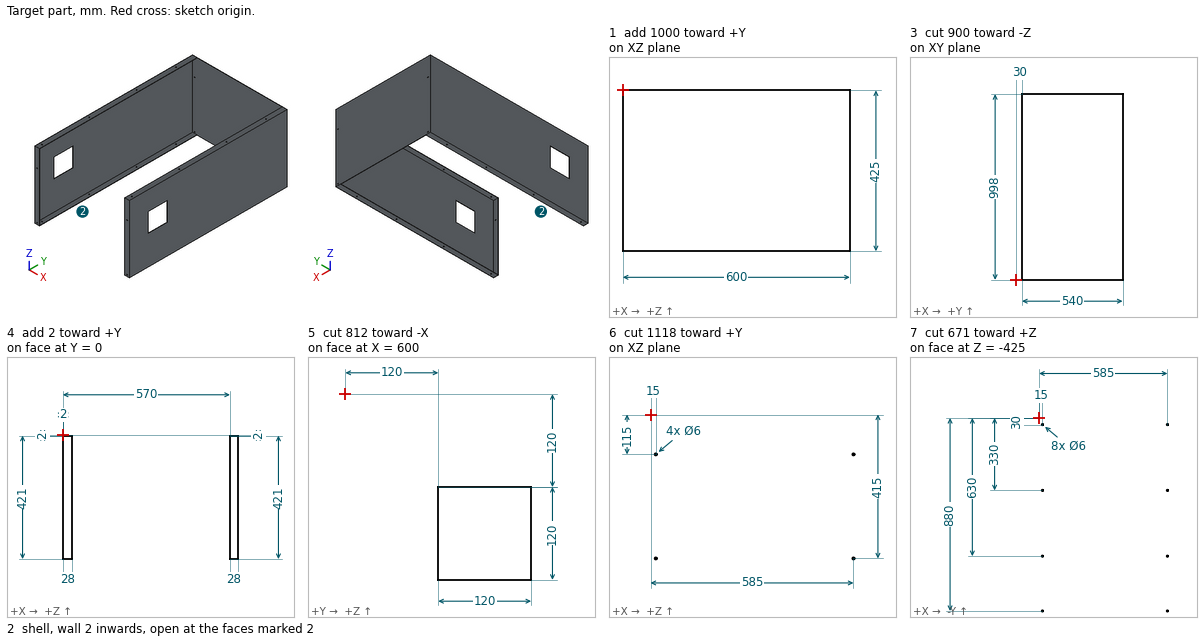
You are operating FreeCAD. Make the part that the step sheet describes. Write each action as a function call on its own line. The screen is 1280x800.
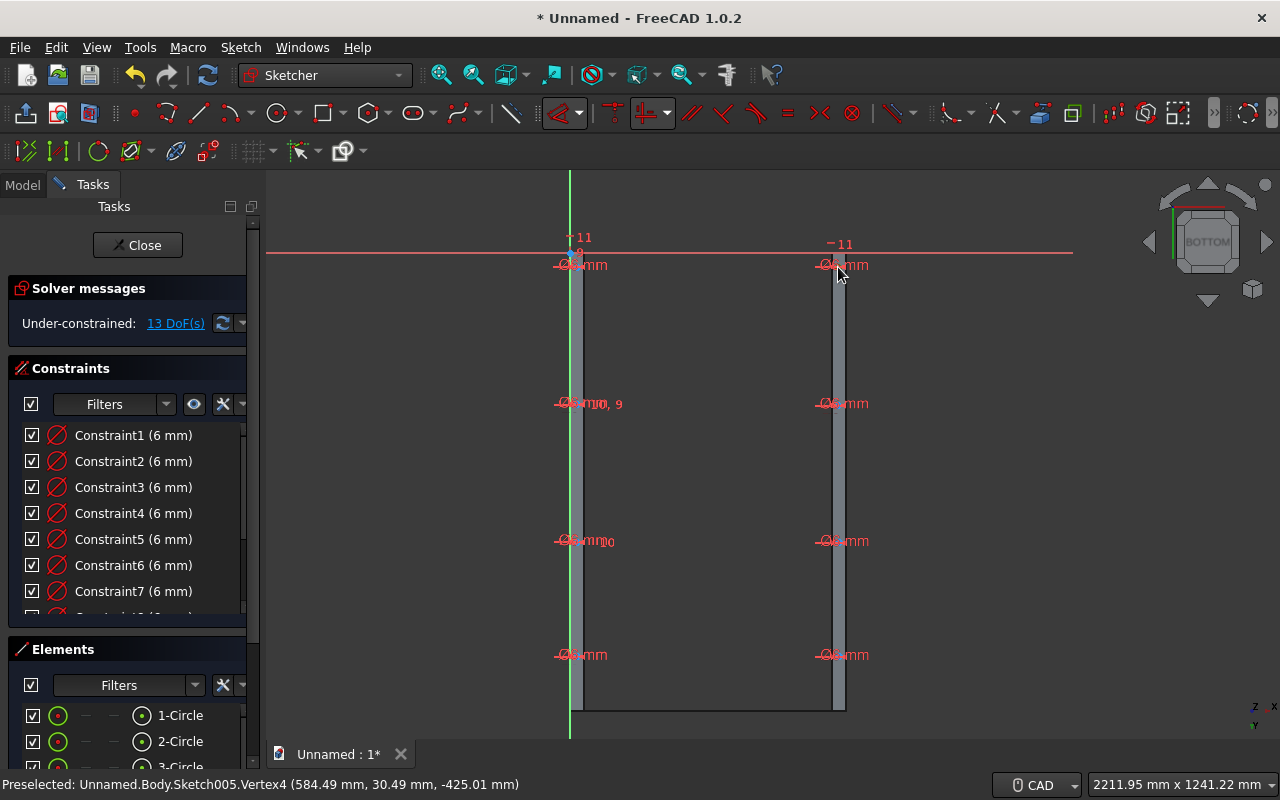
click(838, 406)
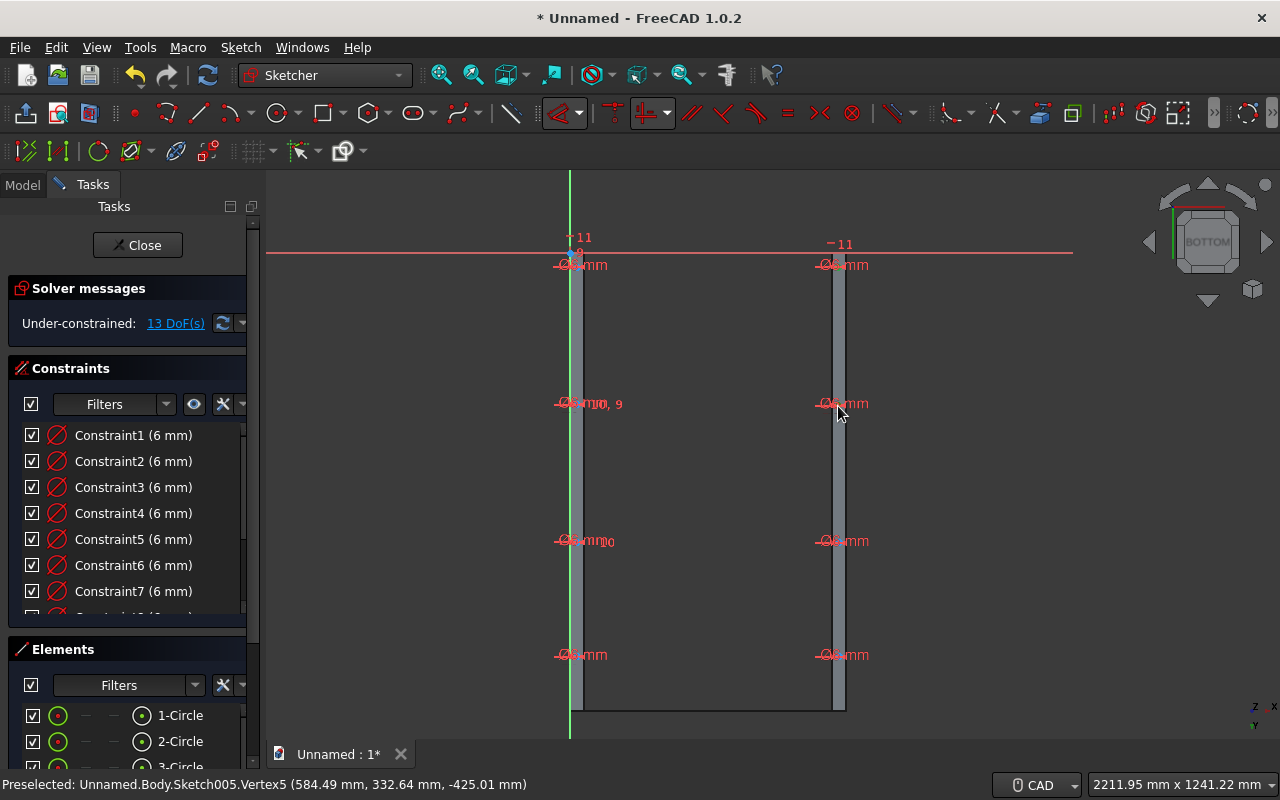
key(v)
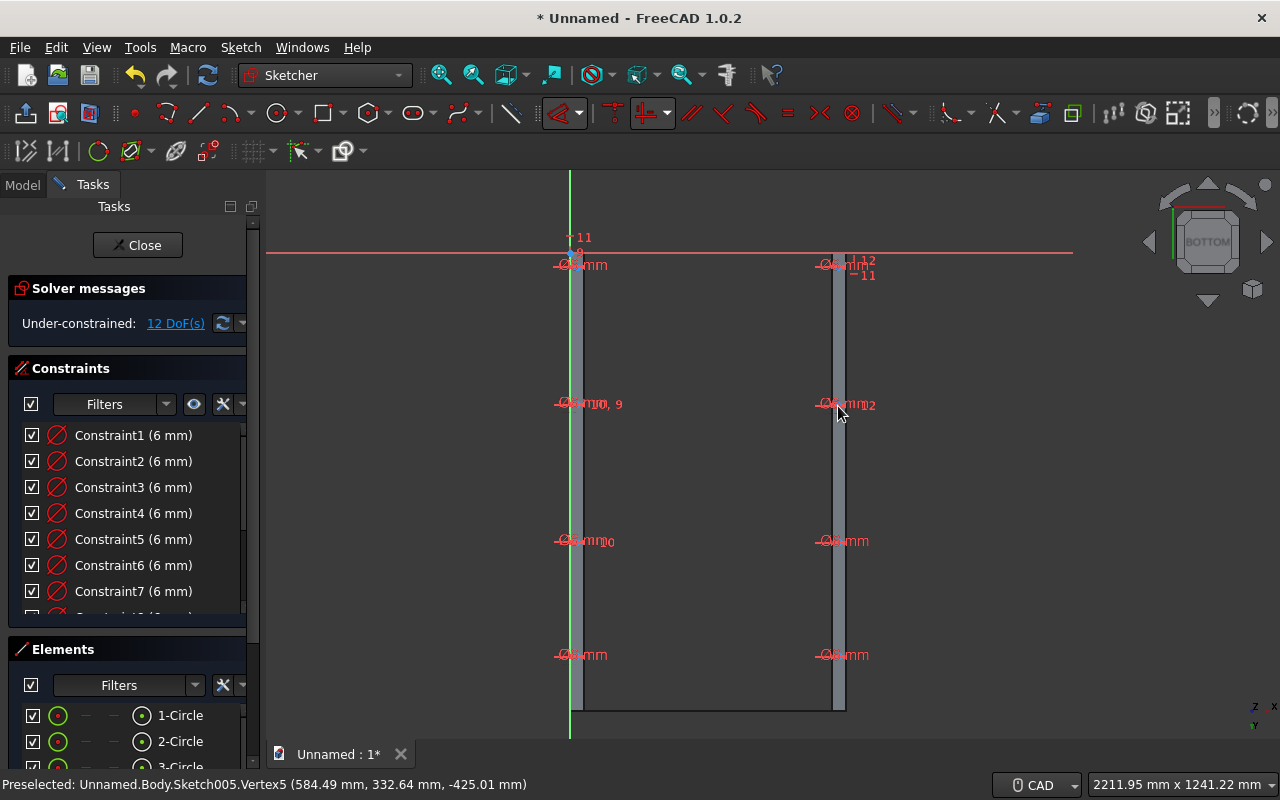
click(577, 405)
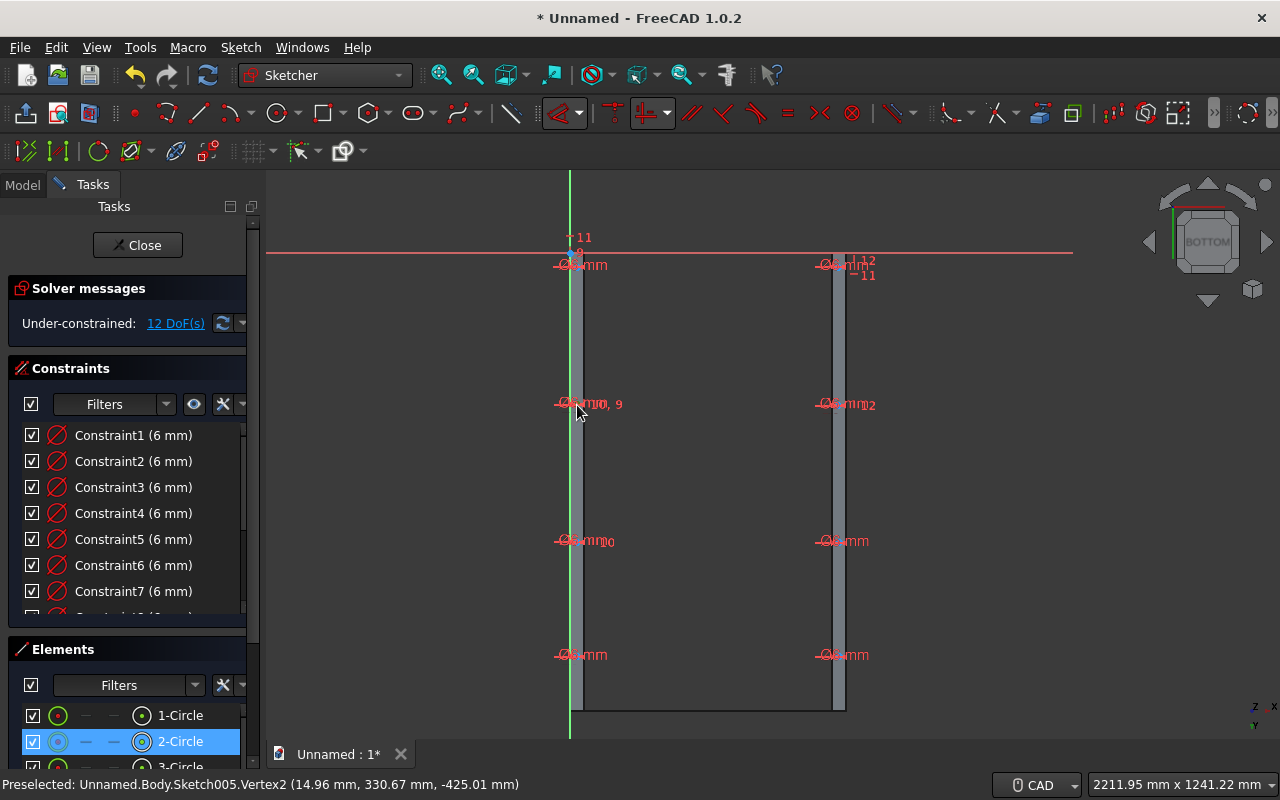
click(838, 406)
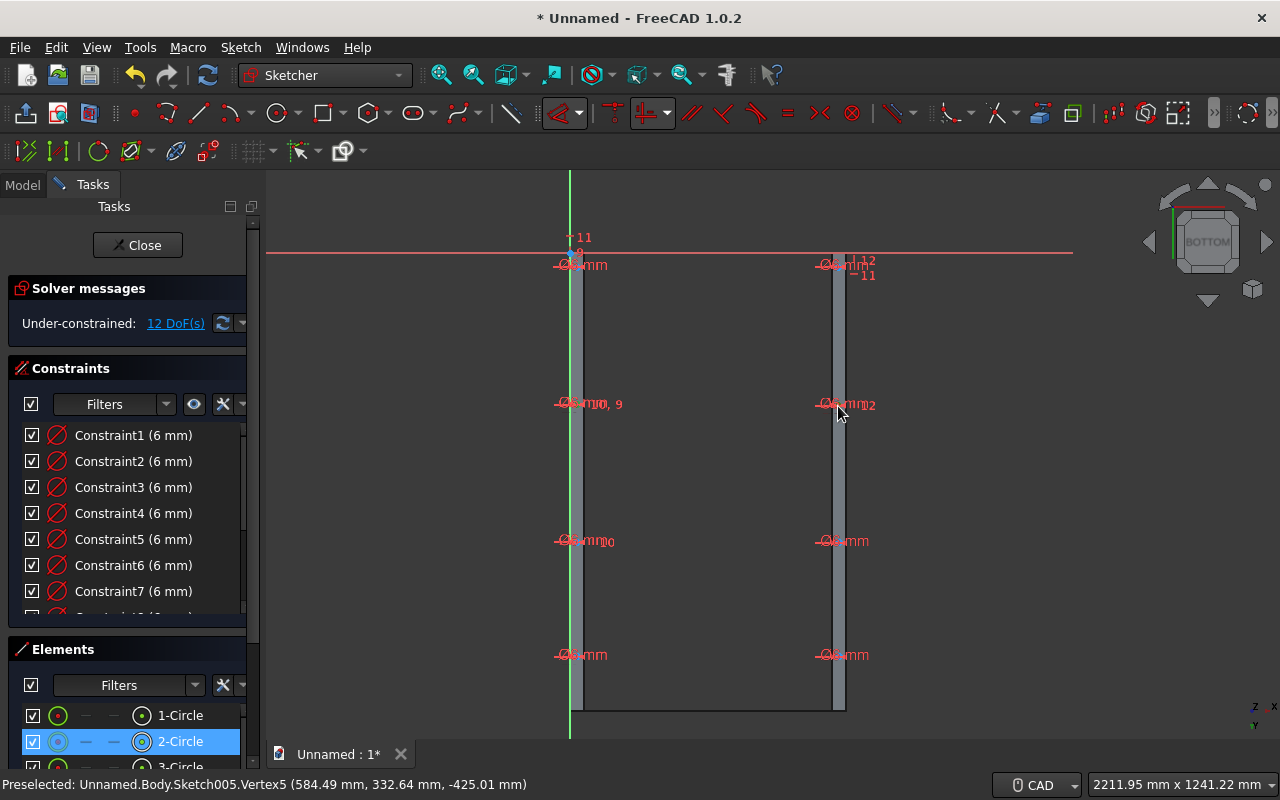
click(670, 114)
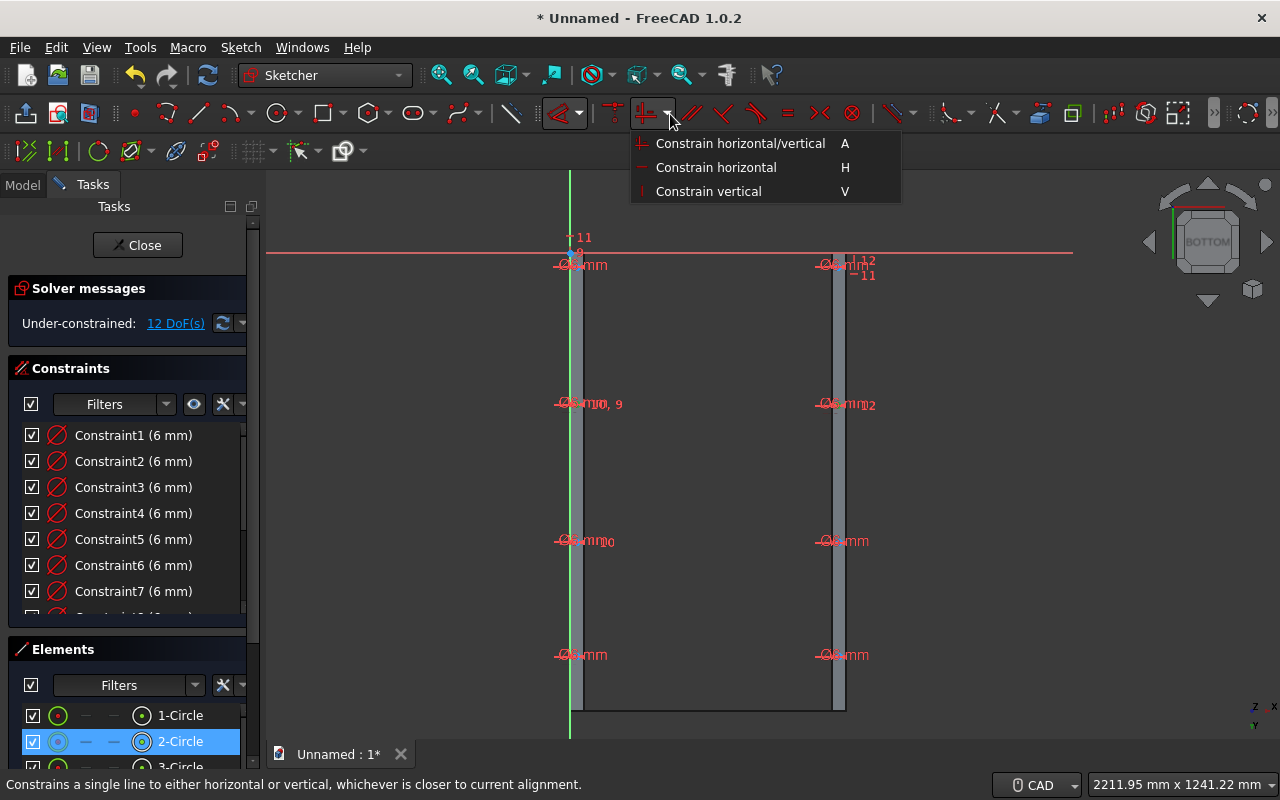
click(766, 167)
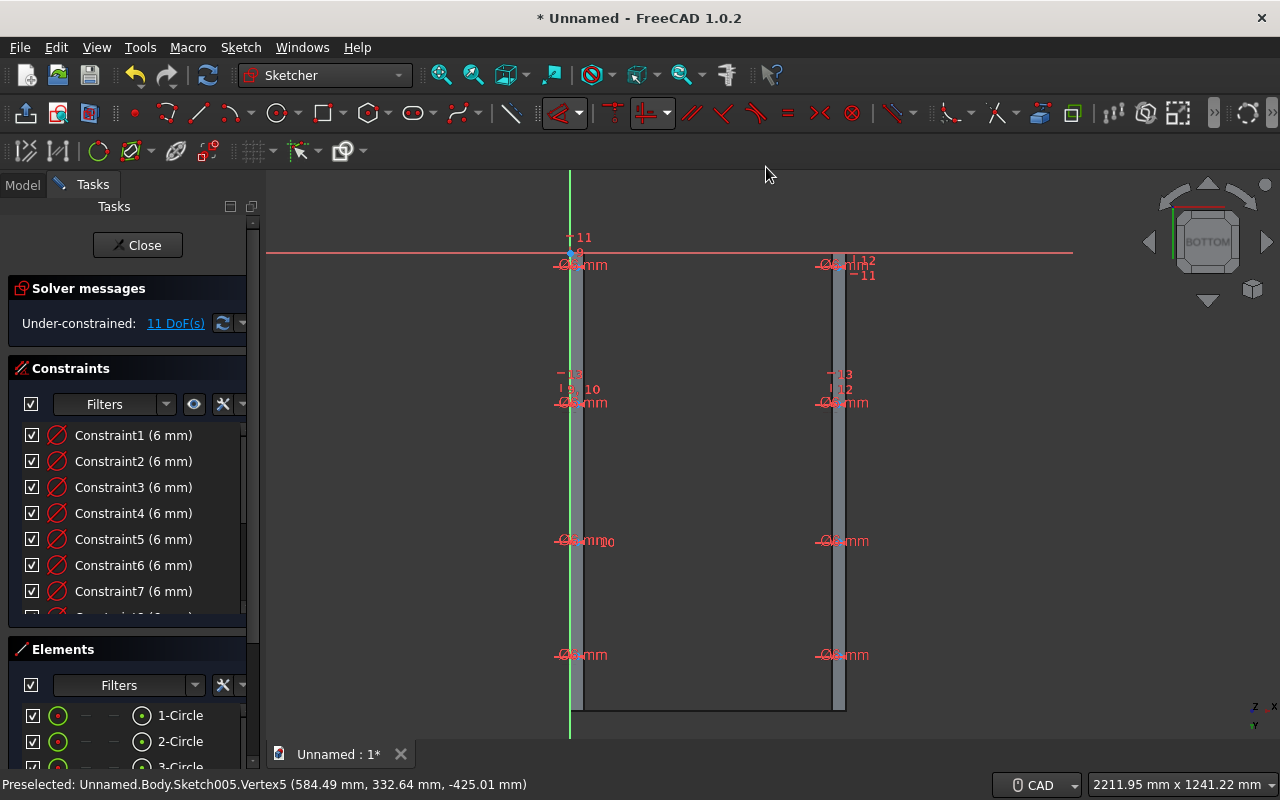
click(577, 542)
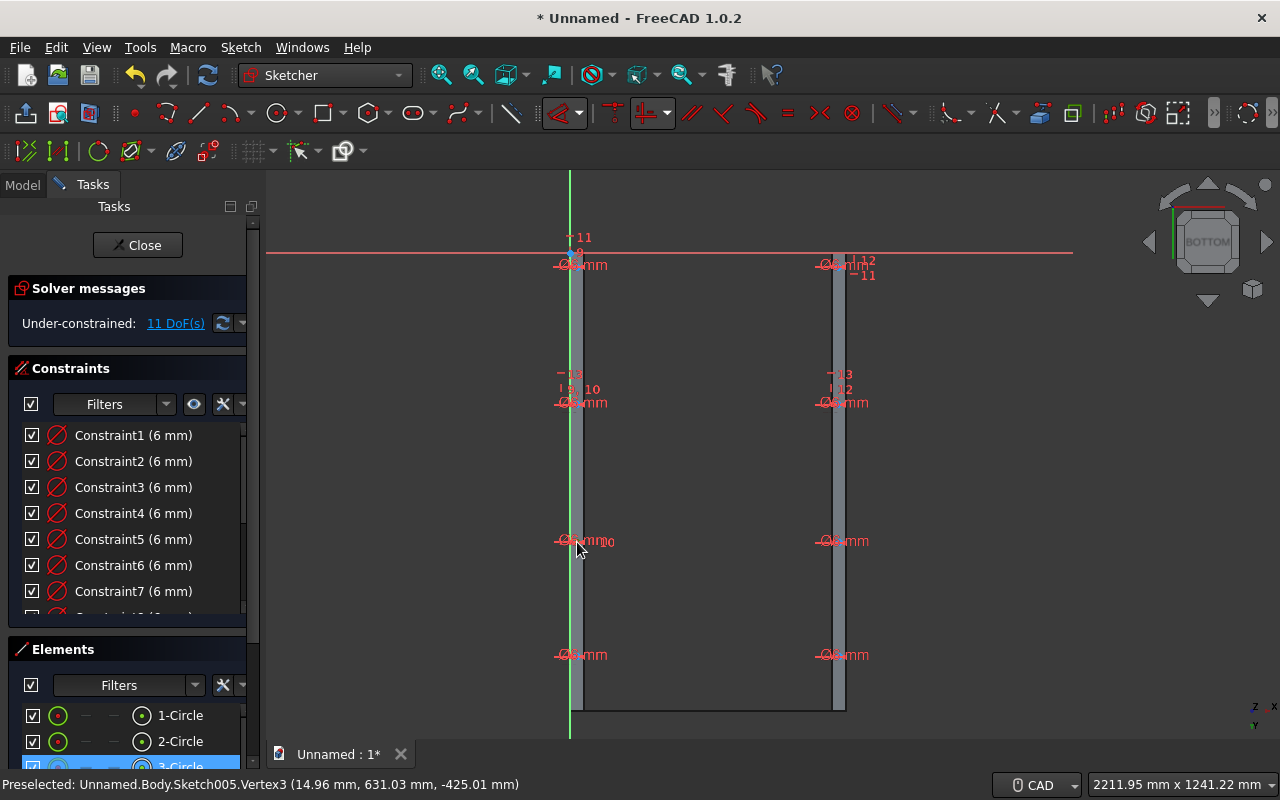
click(577, 657)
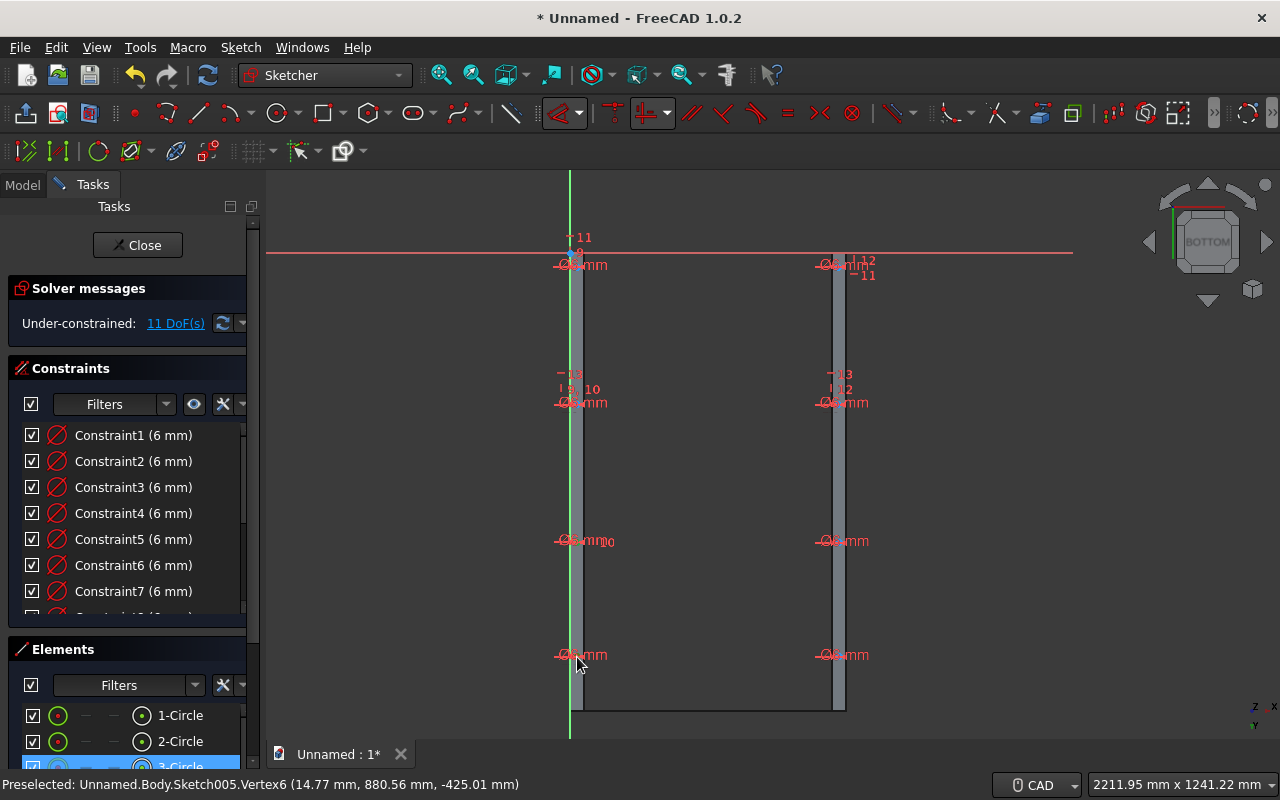
click(670, 114)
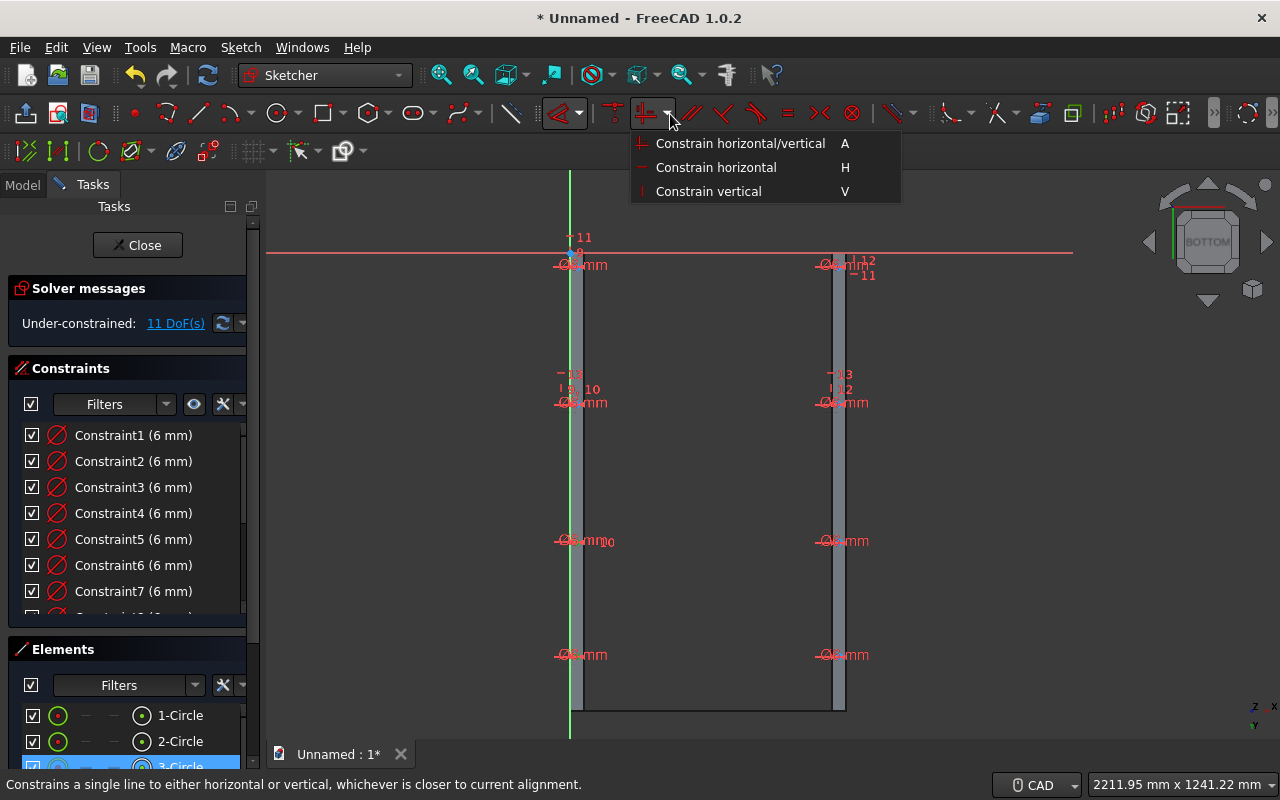
click(766, 191)